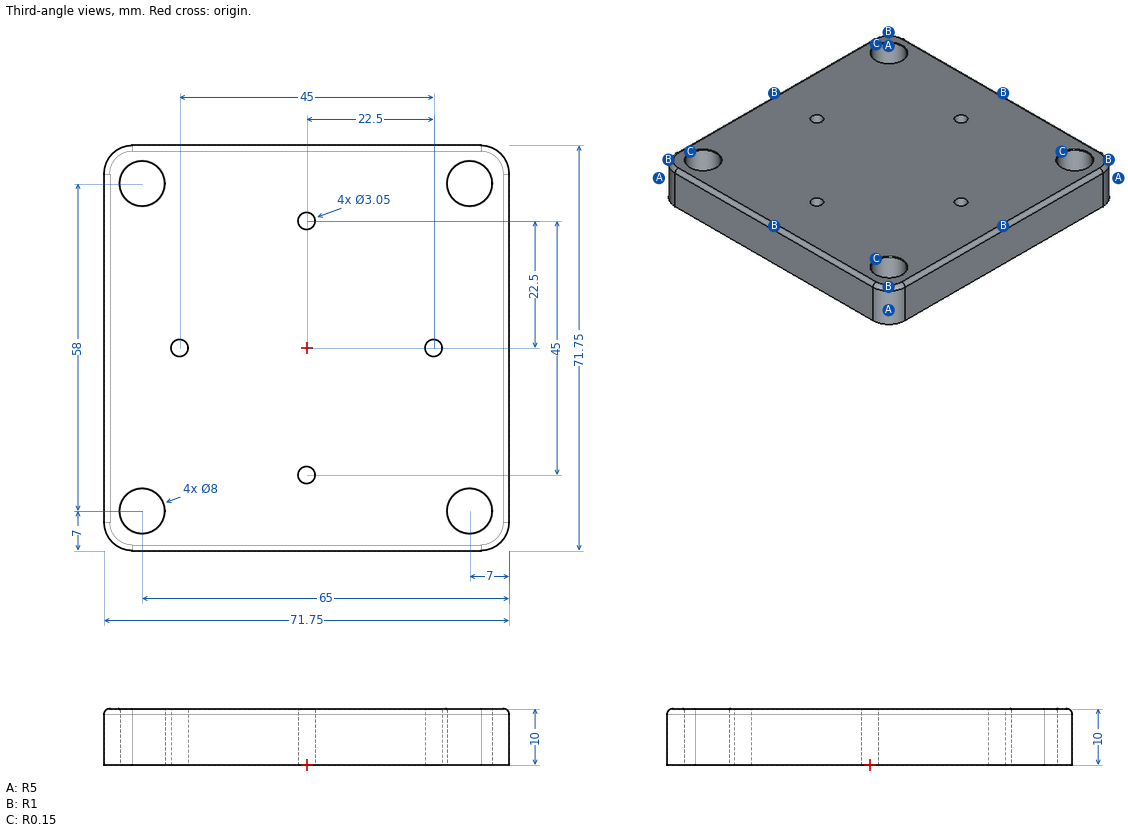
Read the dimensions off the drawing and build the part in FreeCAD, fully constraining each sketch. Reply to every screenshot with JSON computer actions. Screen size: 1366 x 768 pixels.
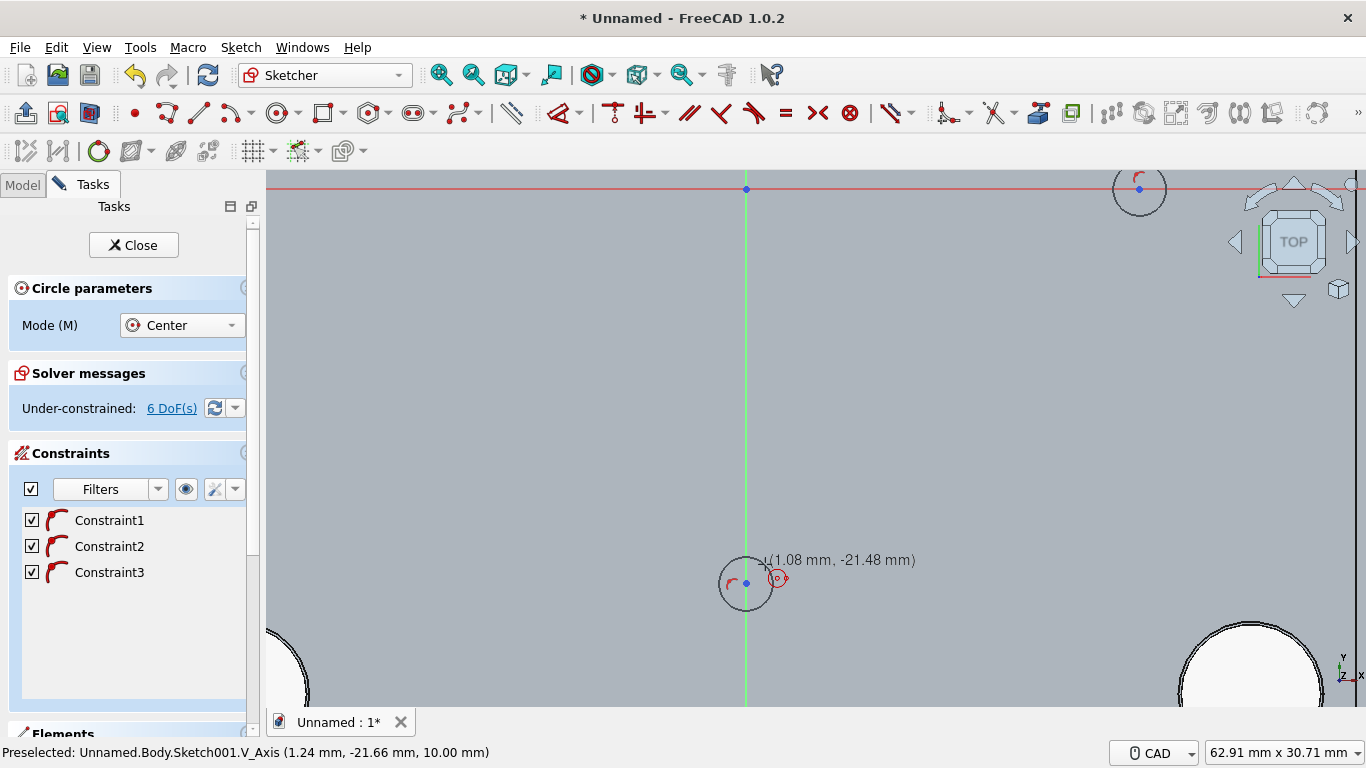
{"action": "scroll", "coordinate": [748, 583], "scroll_direction": "down", "scroll_amount": 5}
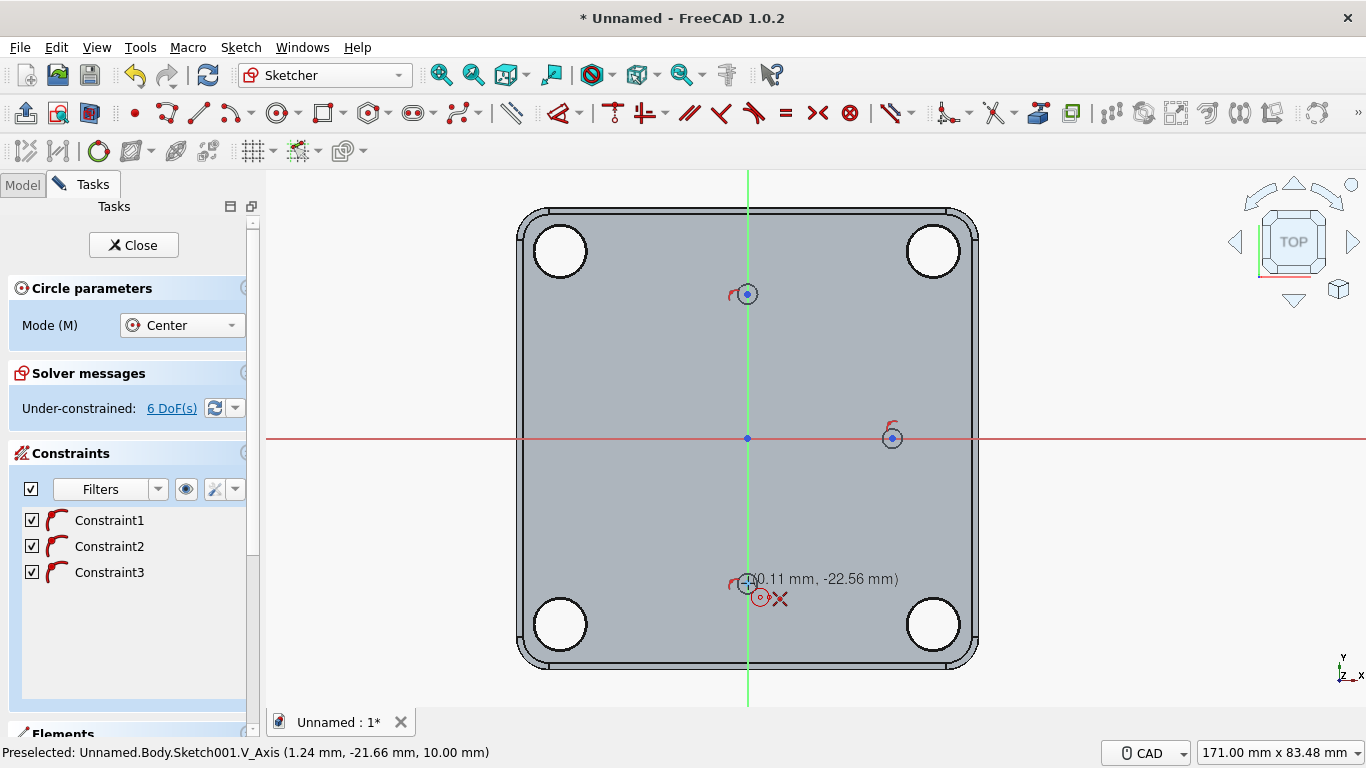
{"action": "scroll", "coordinate": [603, 439], "scroll_direction": "up", "scroll_amount": 5}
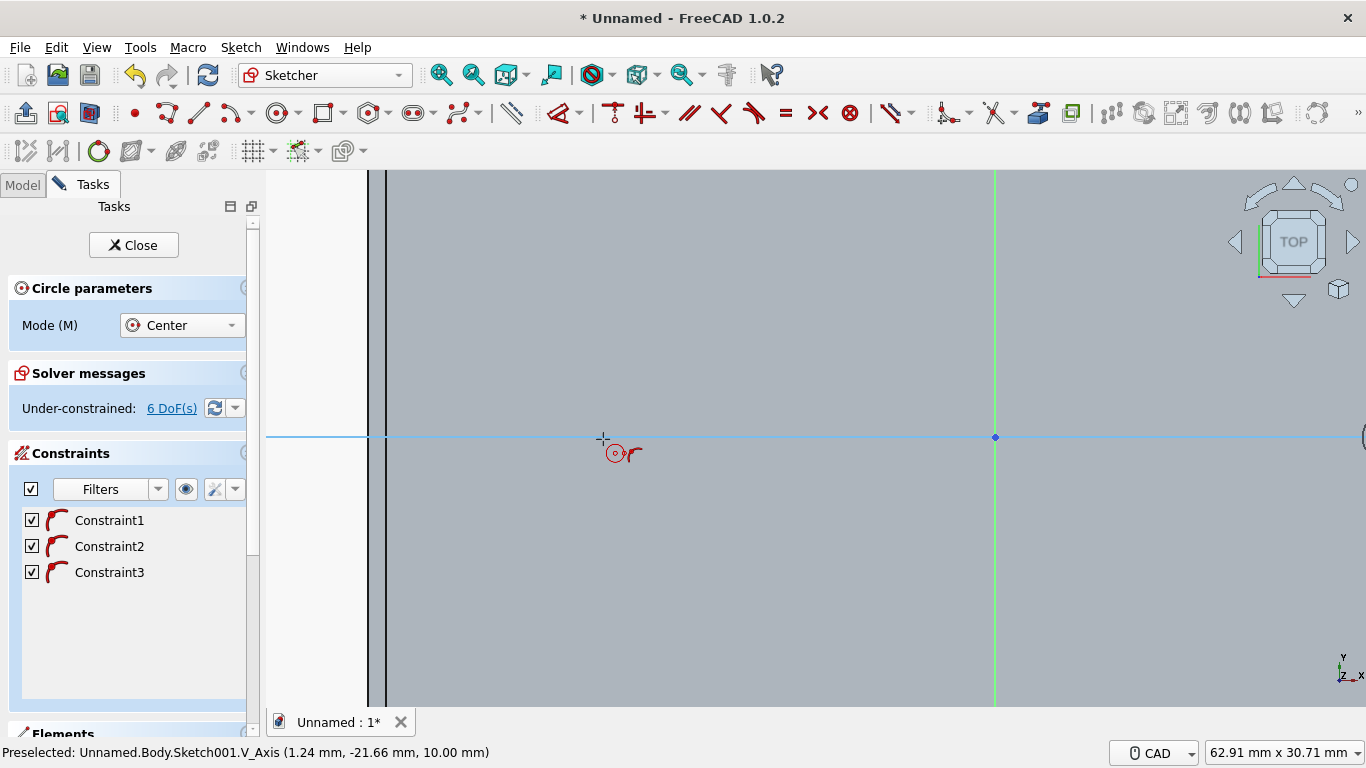
{"action": "left_click", "coordinate": [602, 437]}
{"action": "left_click", "coordinate": [621, 418]}
{"action": "key", "text": "Escape"}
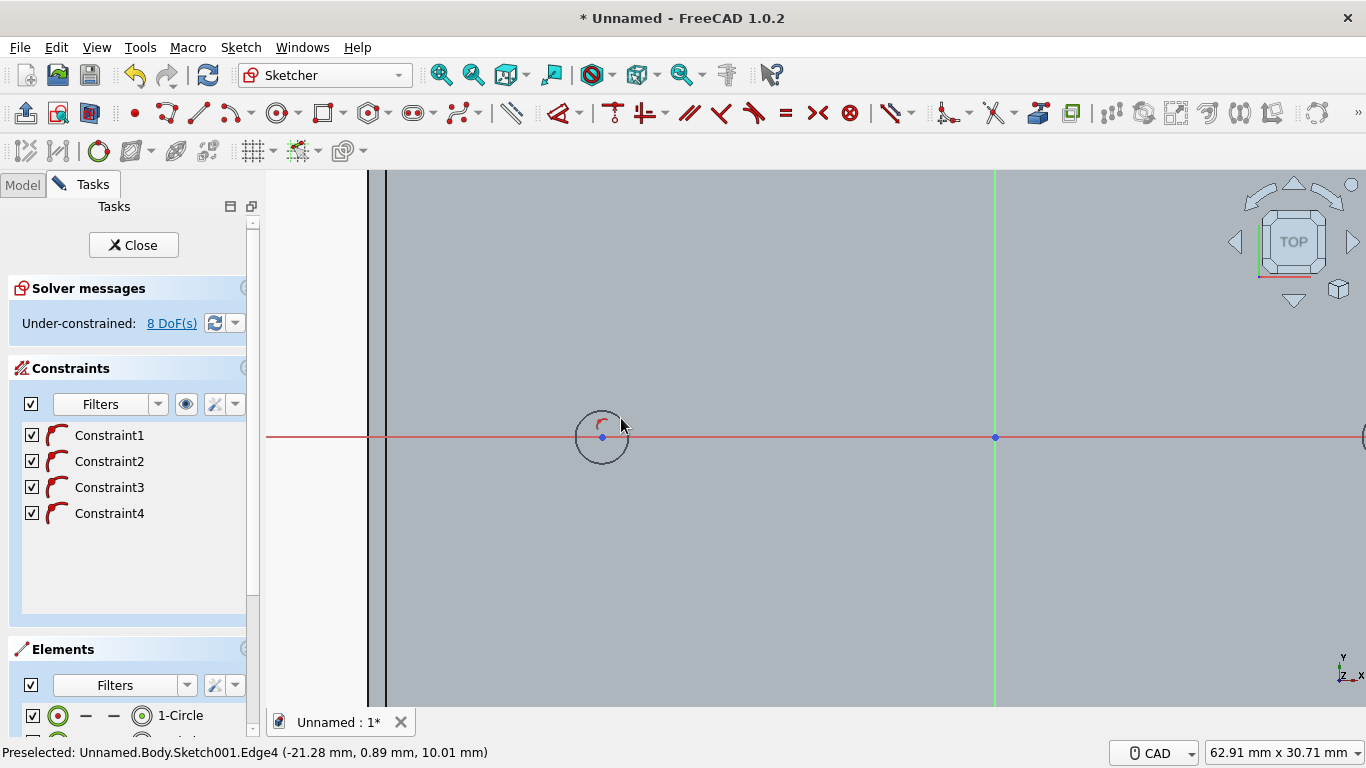
{"action": "scroll", "coordinate": [603, 439], "scroll_direction": "down", "scroll_amount": 5}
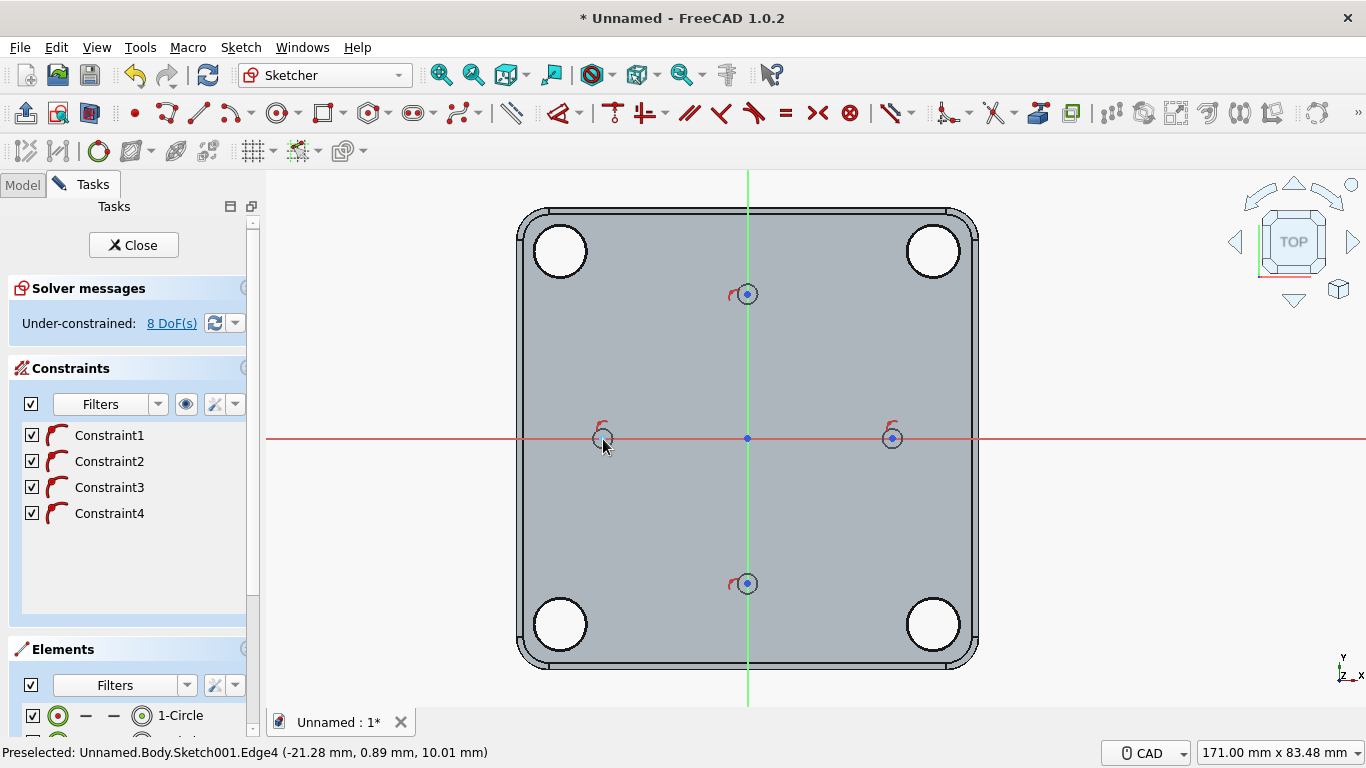
{"action": "scroll", "coordinate": [755, 287], "scroll_direction": "up", "scroll_amount": 4}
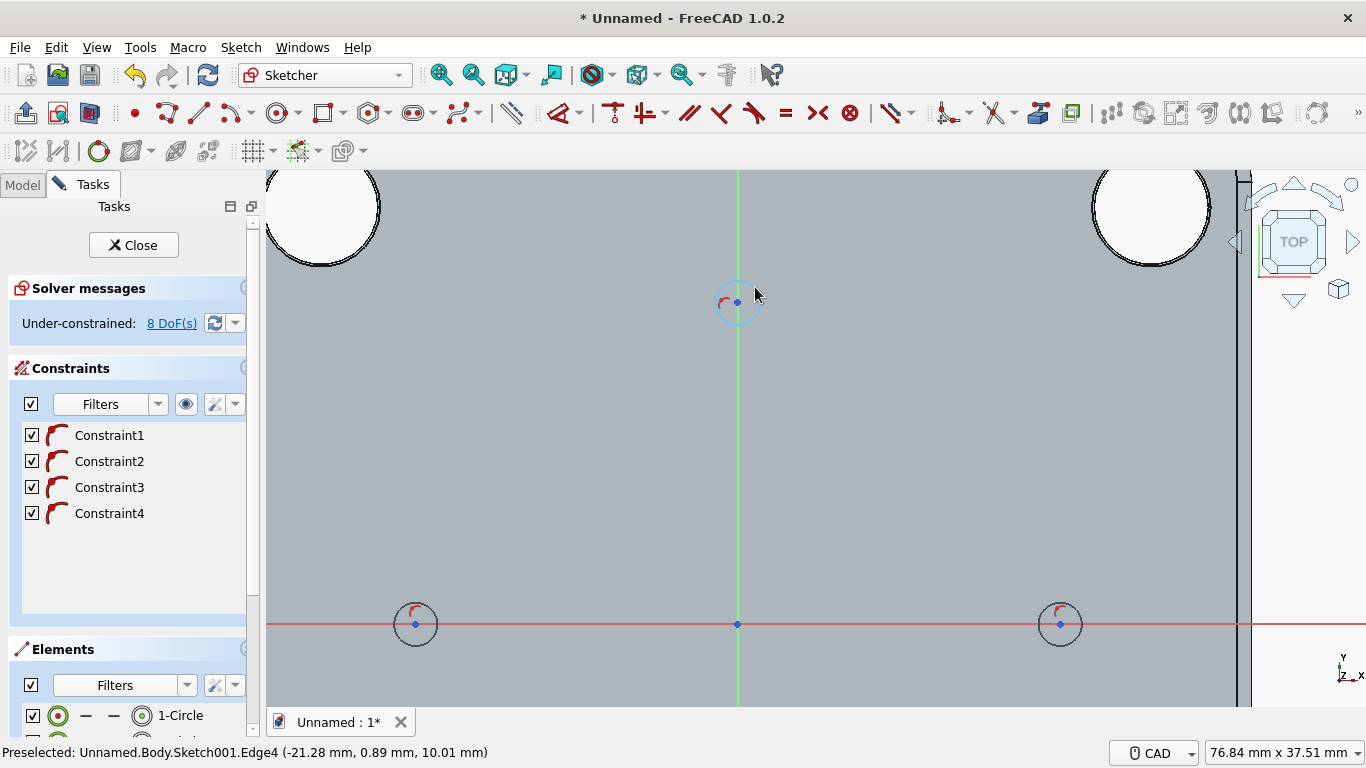
{"action": "left_click", "coordinate": [753, 287]}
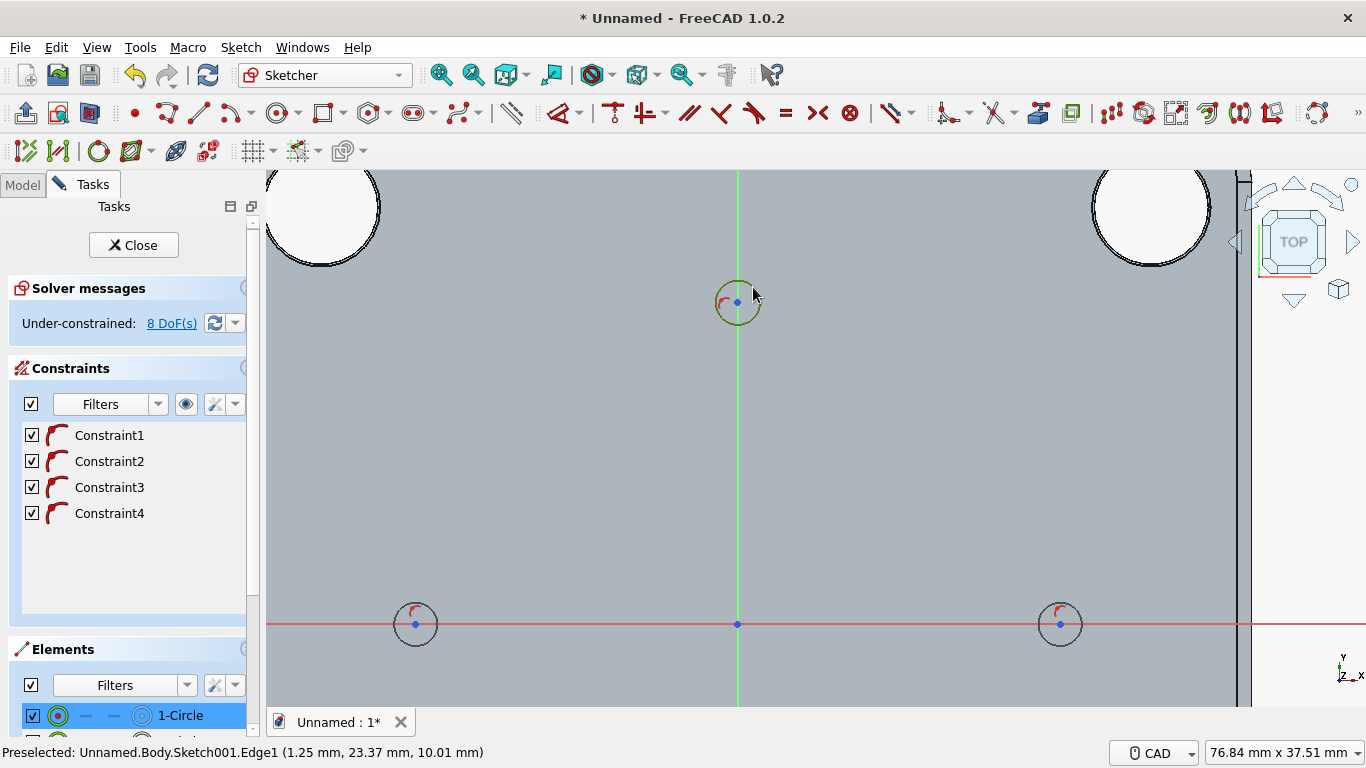
{"action": "left_click", "coordinate": [1075, 609]}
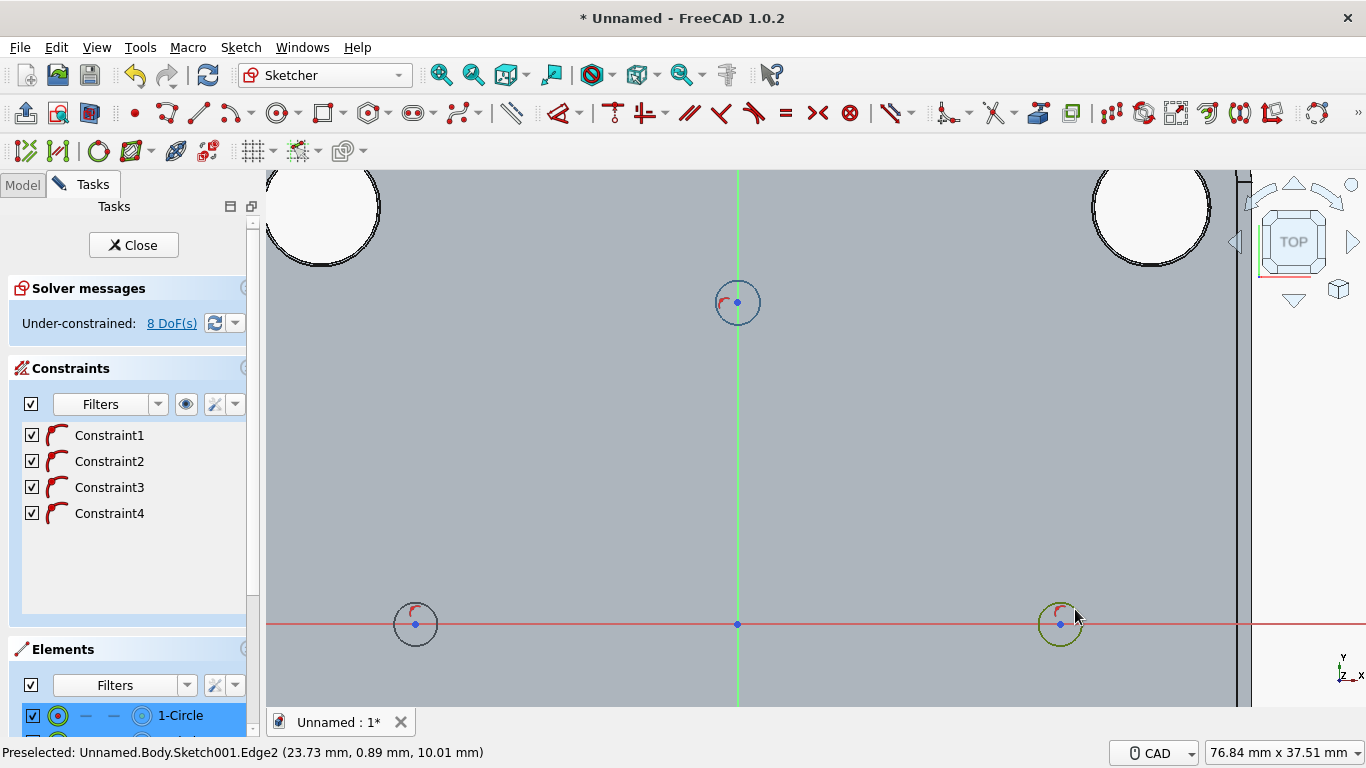
{"action": "scroll", "coordinate": [755, 287], "scroll_direction": "down", "scroll_amount": 4}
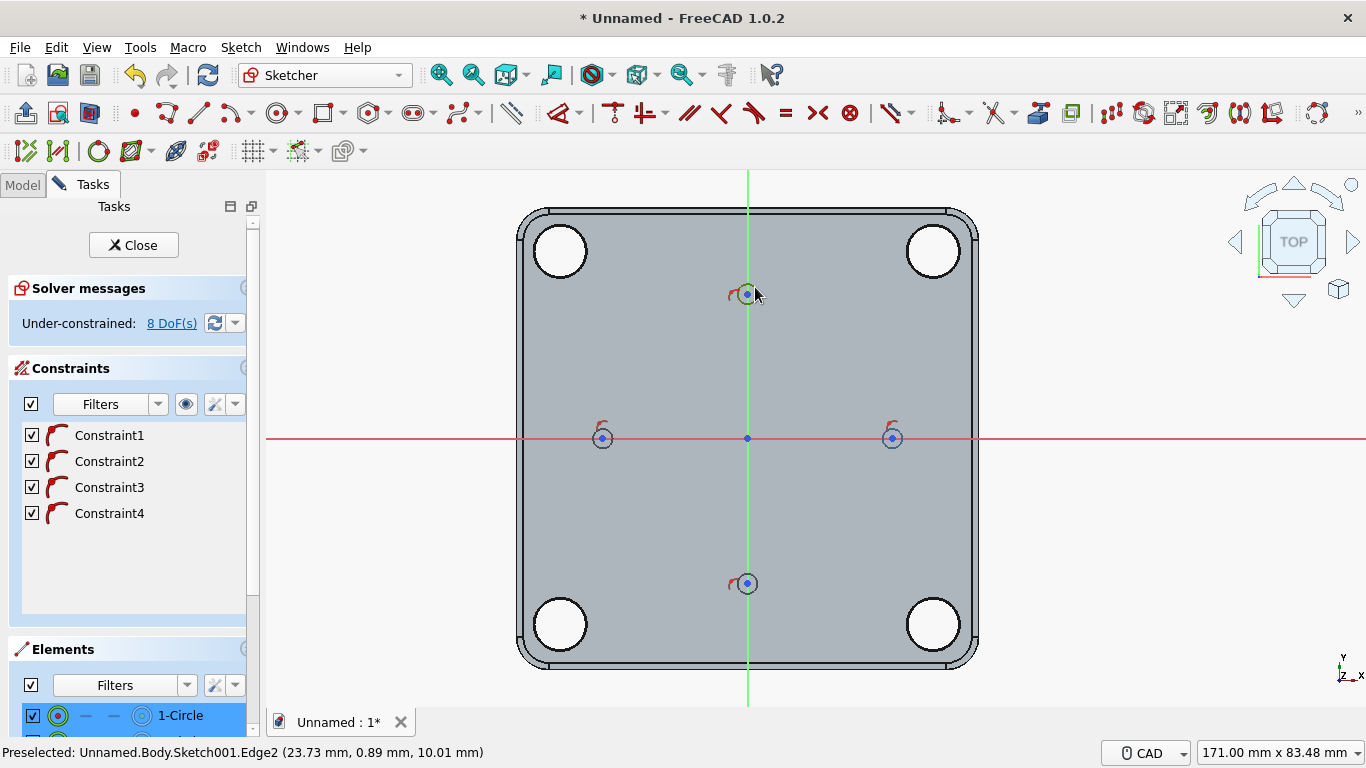
{"action": "scroll", "coordinate": [755, 577], "scroll_direction": "up", "scroll_amount": 4}